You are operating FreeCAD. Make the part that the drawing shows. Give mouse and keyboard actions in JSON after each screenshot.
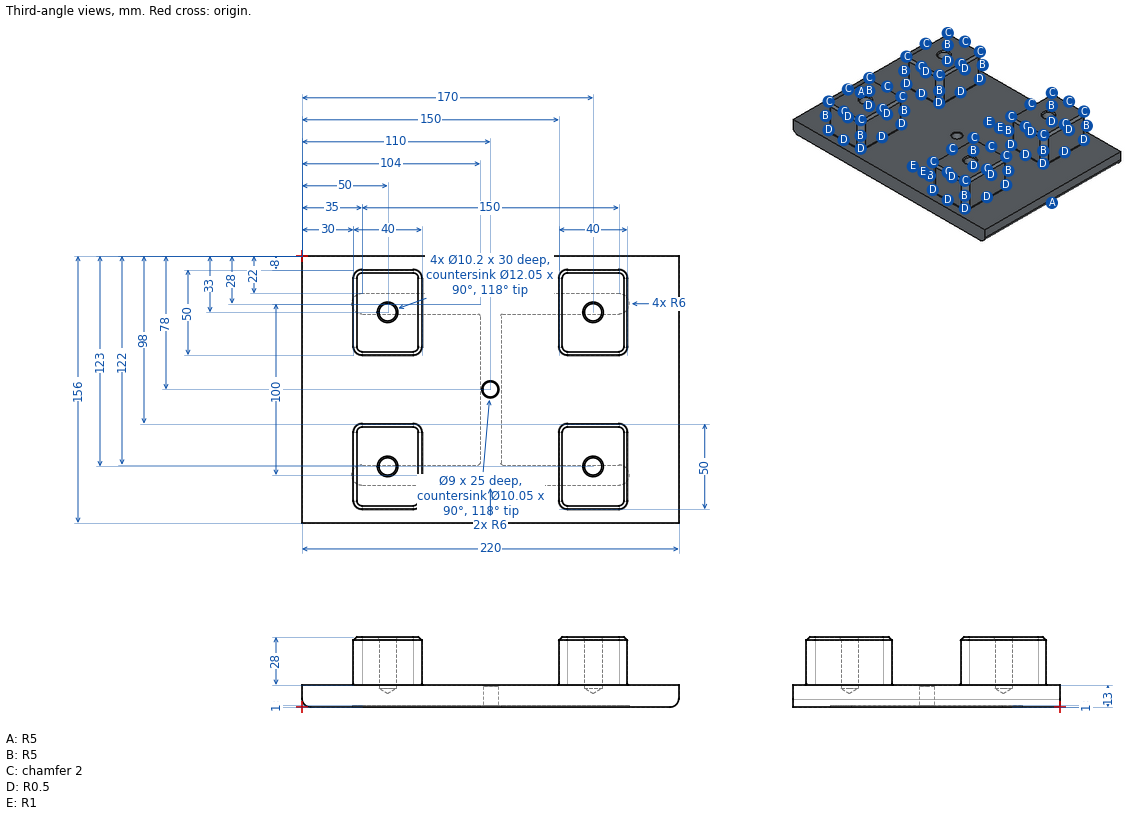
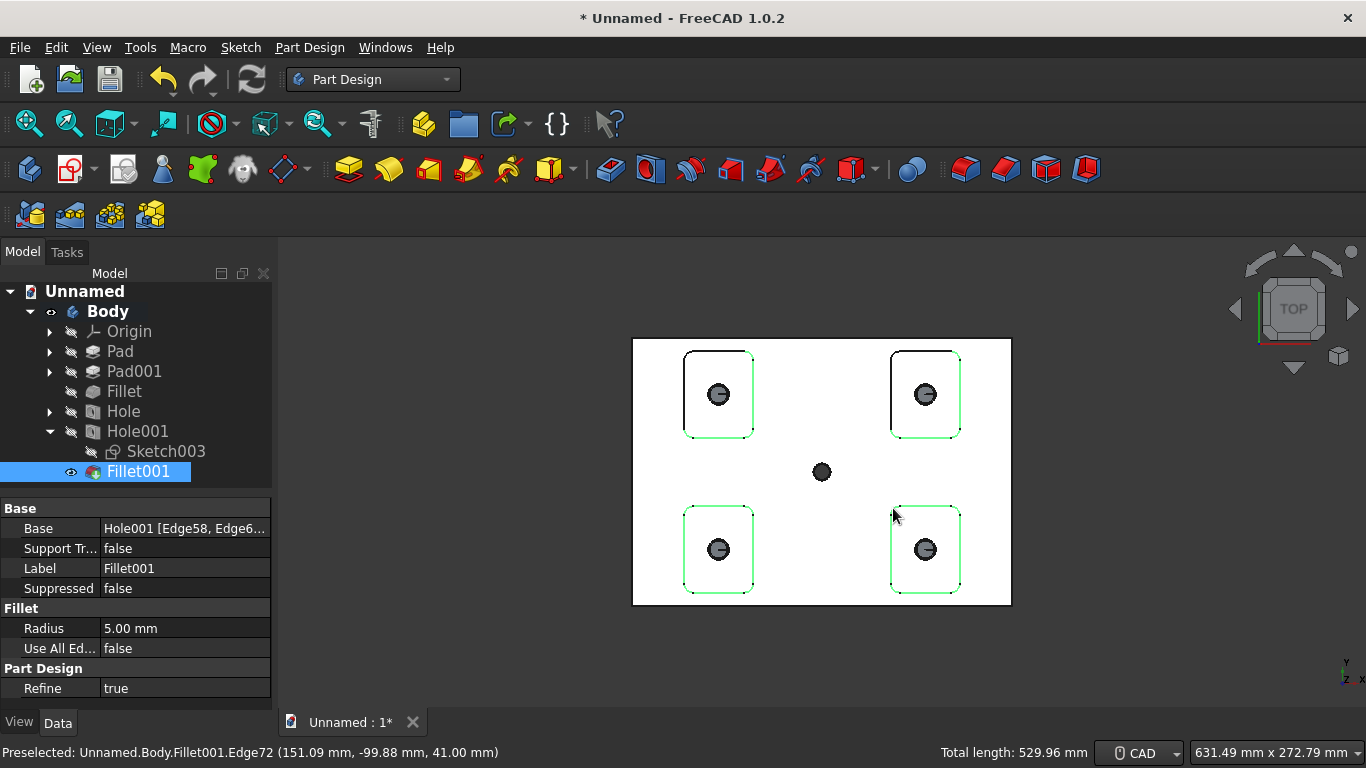
{"action": "left_click", "coordinate": [891, 393], "text": "ctrl"}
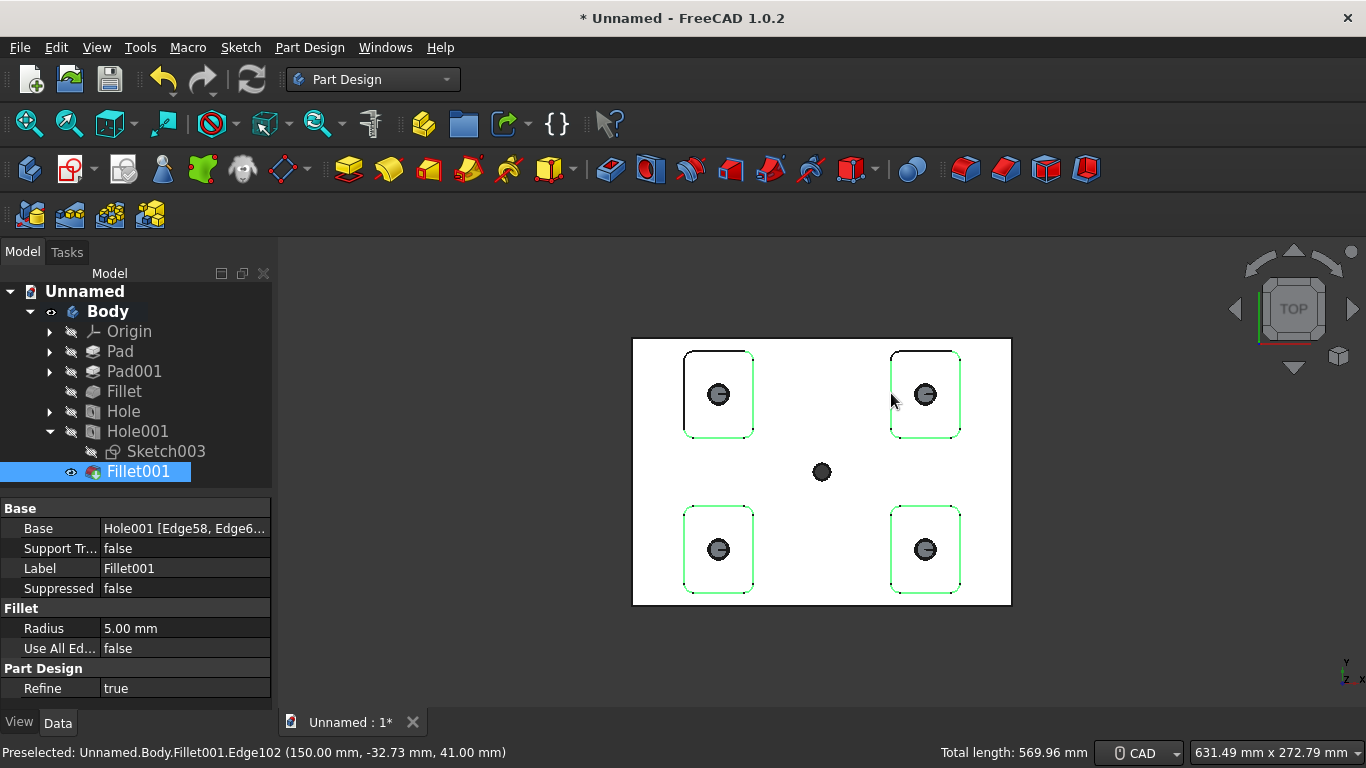
{"action": "left_click", "coordinate": [925, 350], "text": "ctrl"}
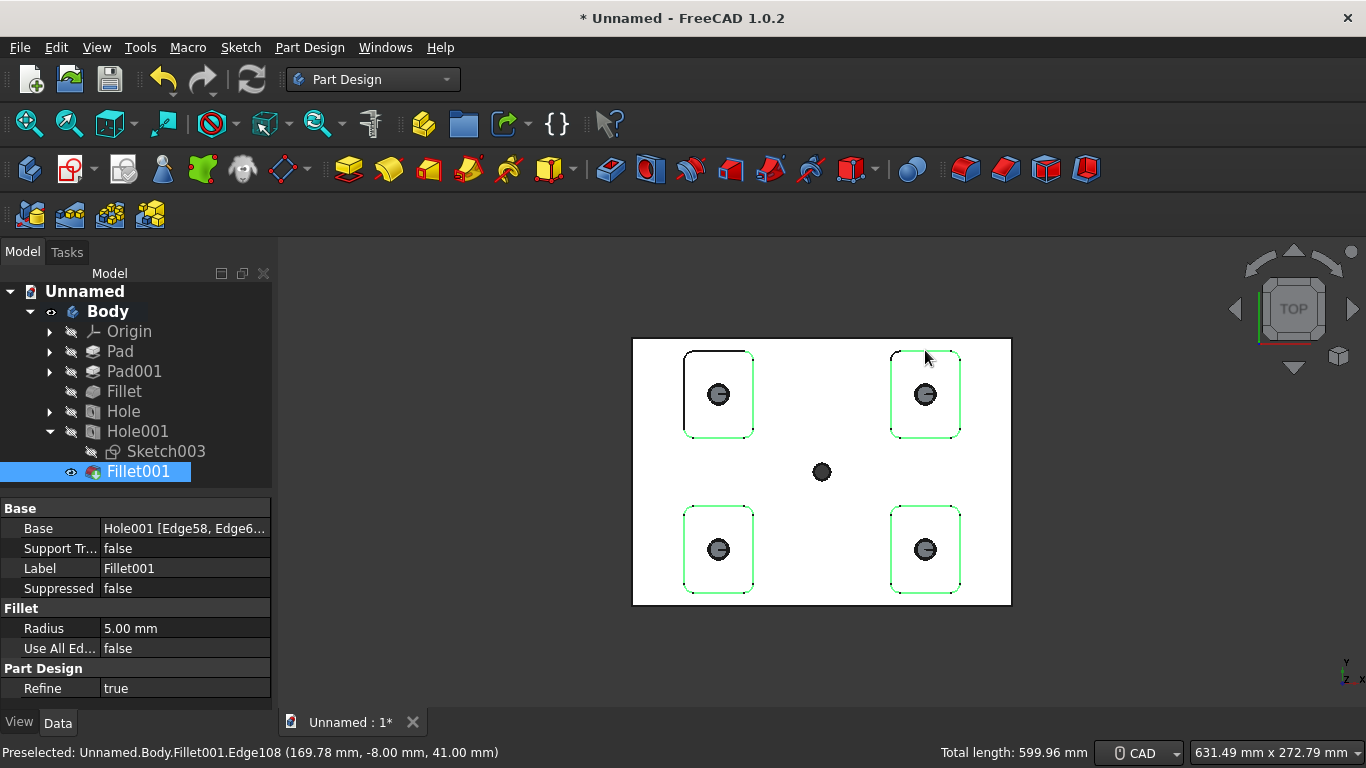
{"action": "left_click", "coordinate": [893, 353], "text": "ctrl"}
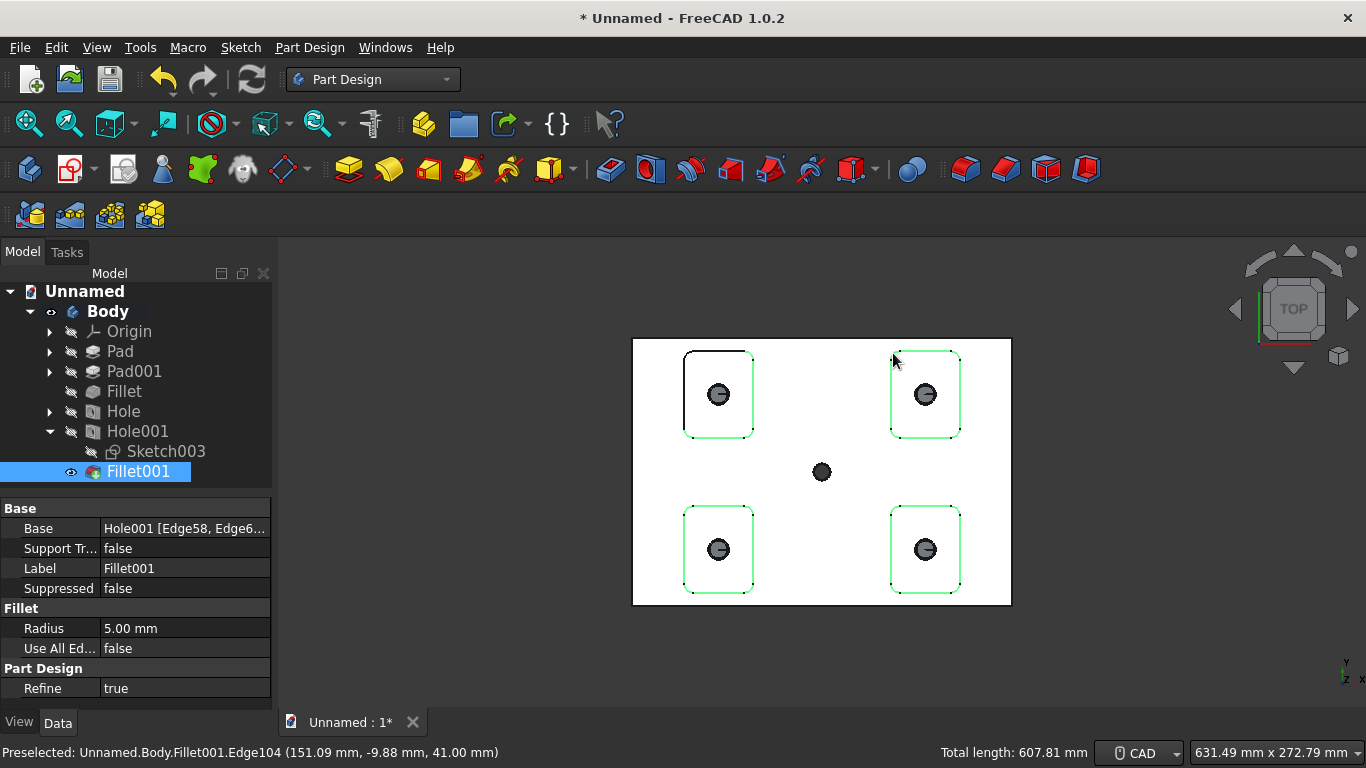
{"action": "left_click", "coordinate": [719, 350], "text": "ctrl"}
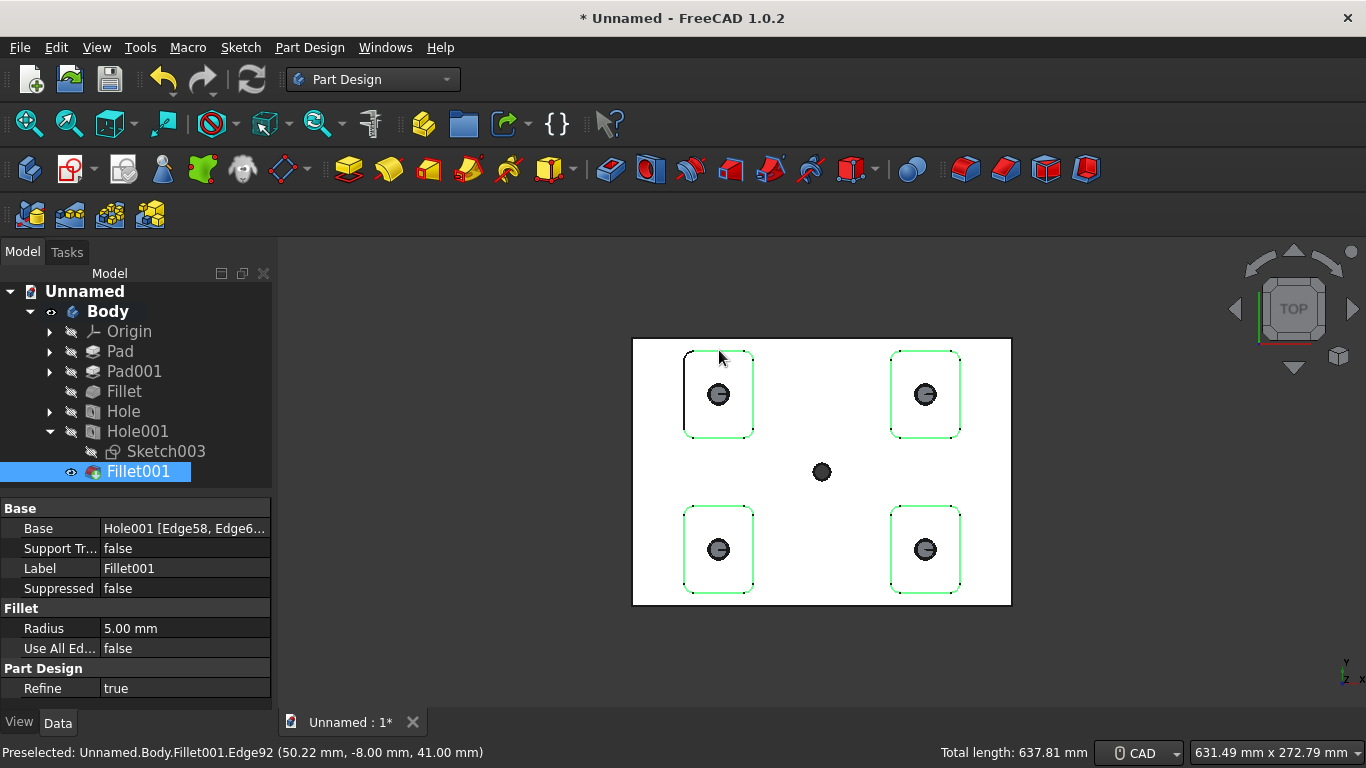
{"action": "left_click", "coordinate": [684, 393], "text": "ctrl"}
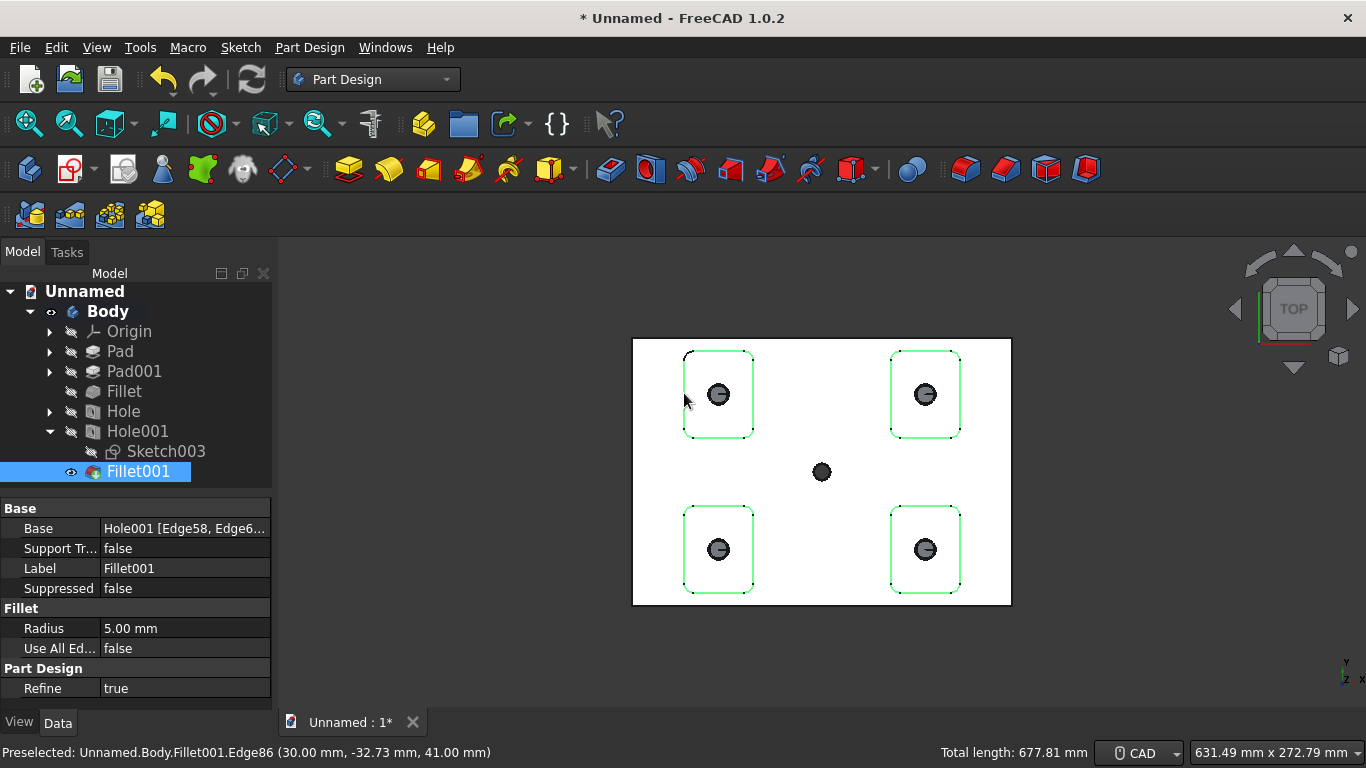
{"action": "left_click", "coordinate": [687, 353], "text": "ctrl"}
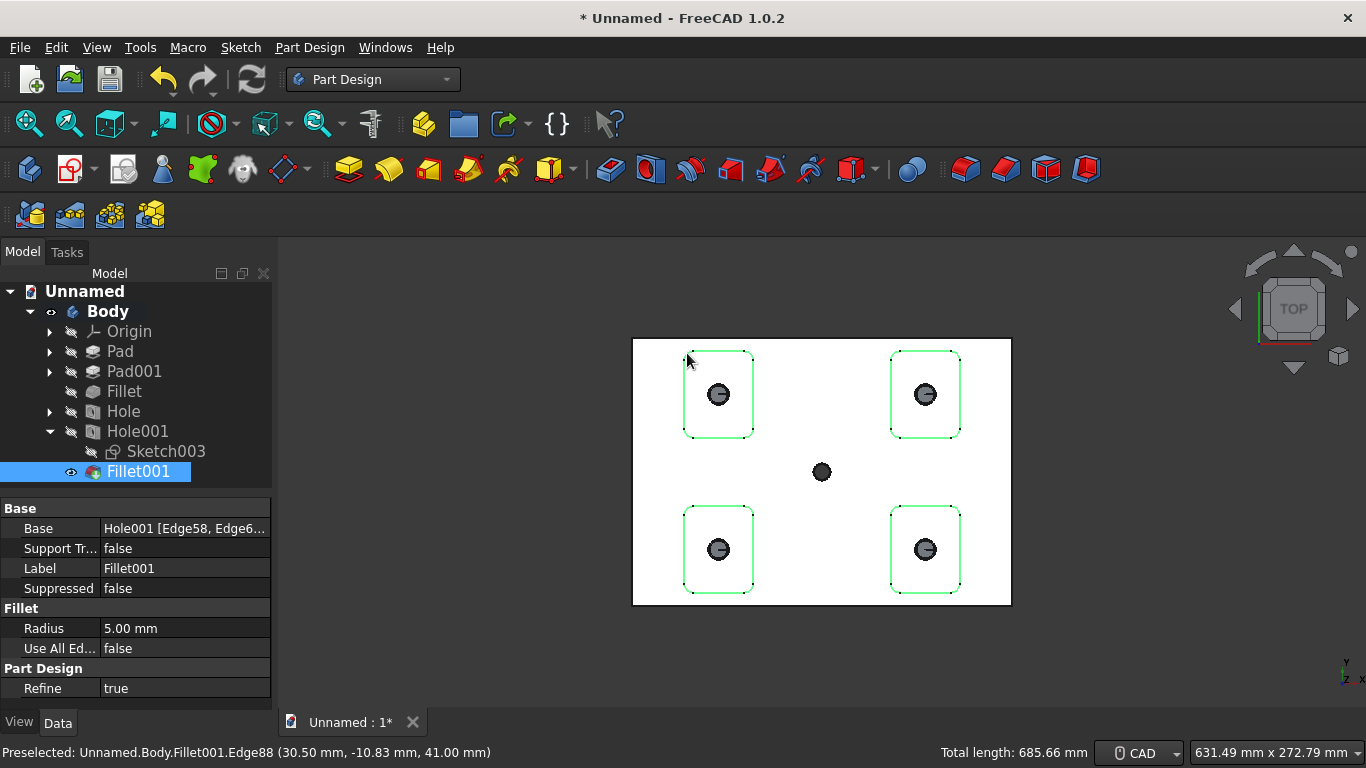
{"action": "left_click", "coordinate": [1006, 170]}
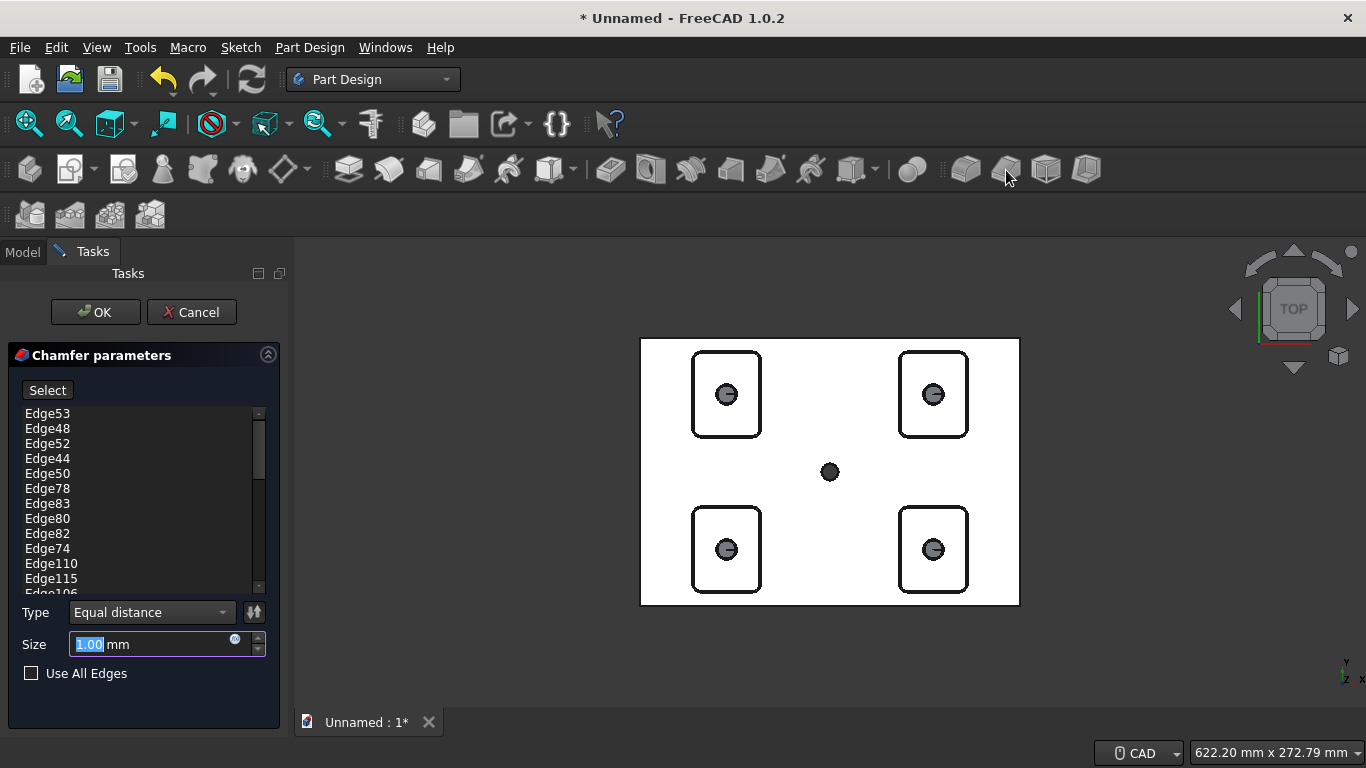
{"action": "type", "text": "2"}
{"action": "key", "text": "Tab"}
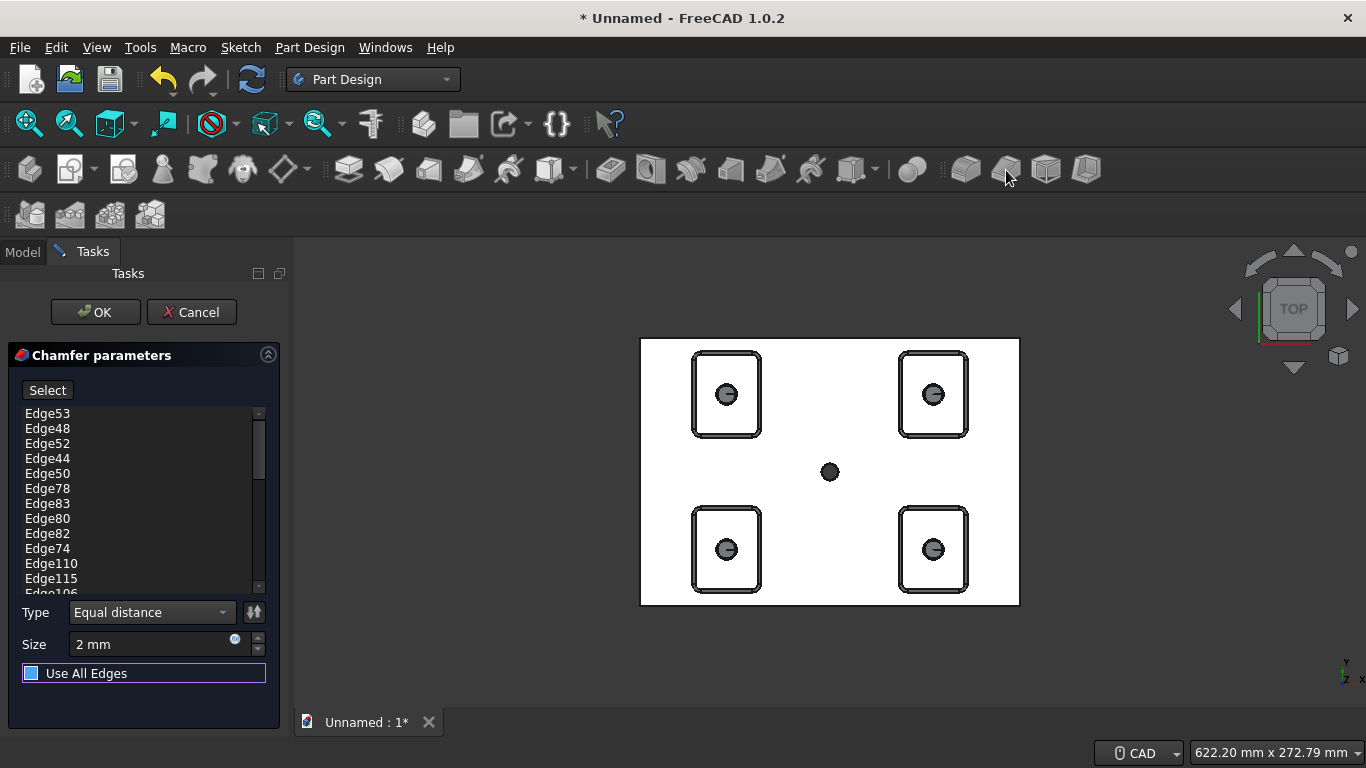
{"action": "left_click", "coordinate": [96, 312]}